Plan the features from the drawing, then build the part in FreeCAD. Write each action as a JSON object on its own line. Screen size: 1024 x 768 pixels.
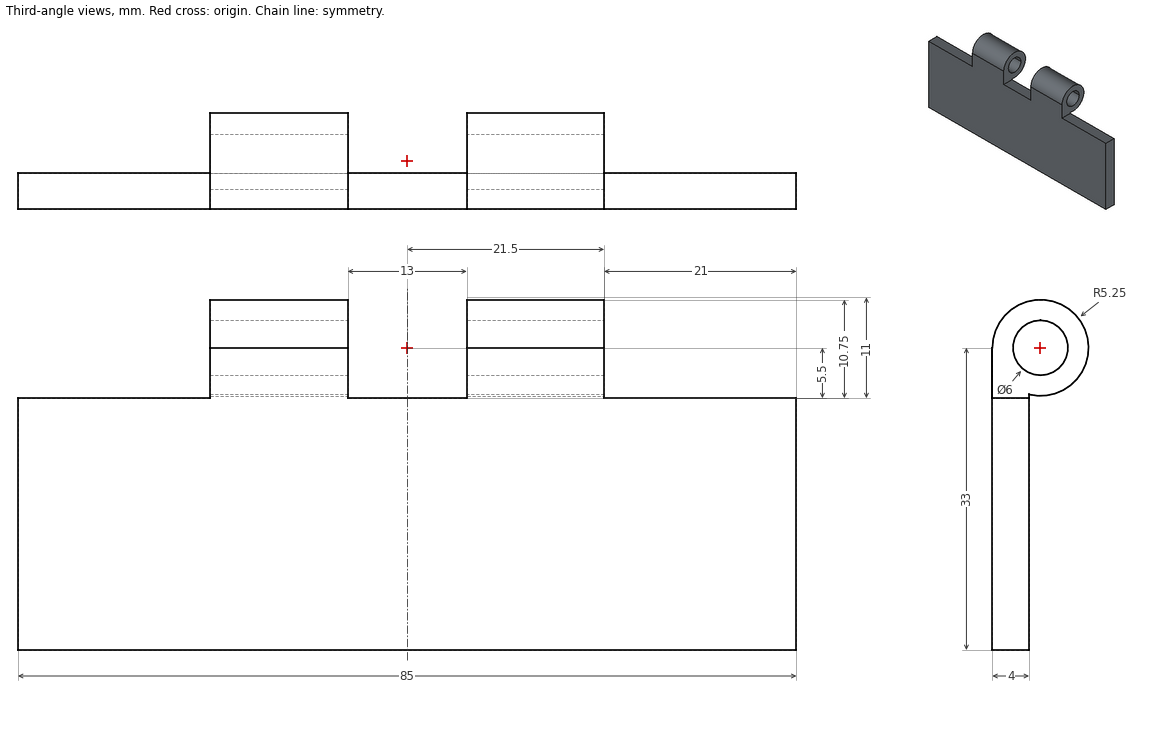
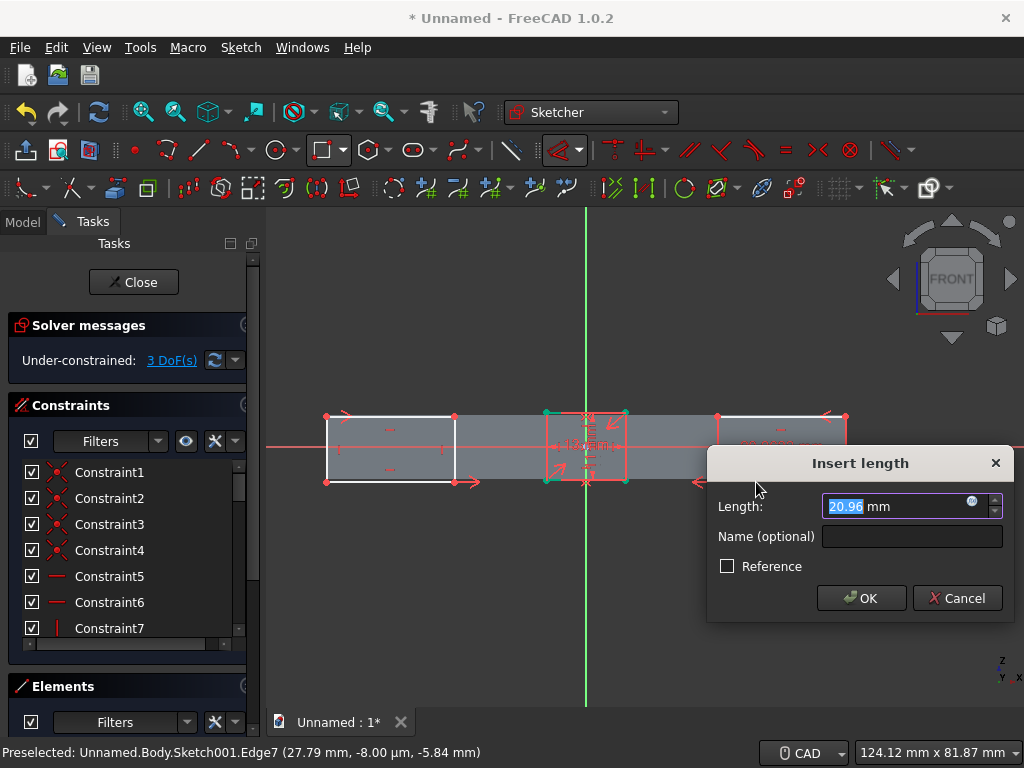
{"action": "type", "text": "21"}
{"action": "key", "text": "Return"}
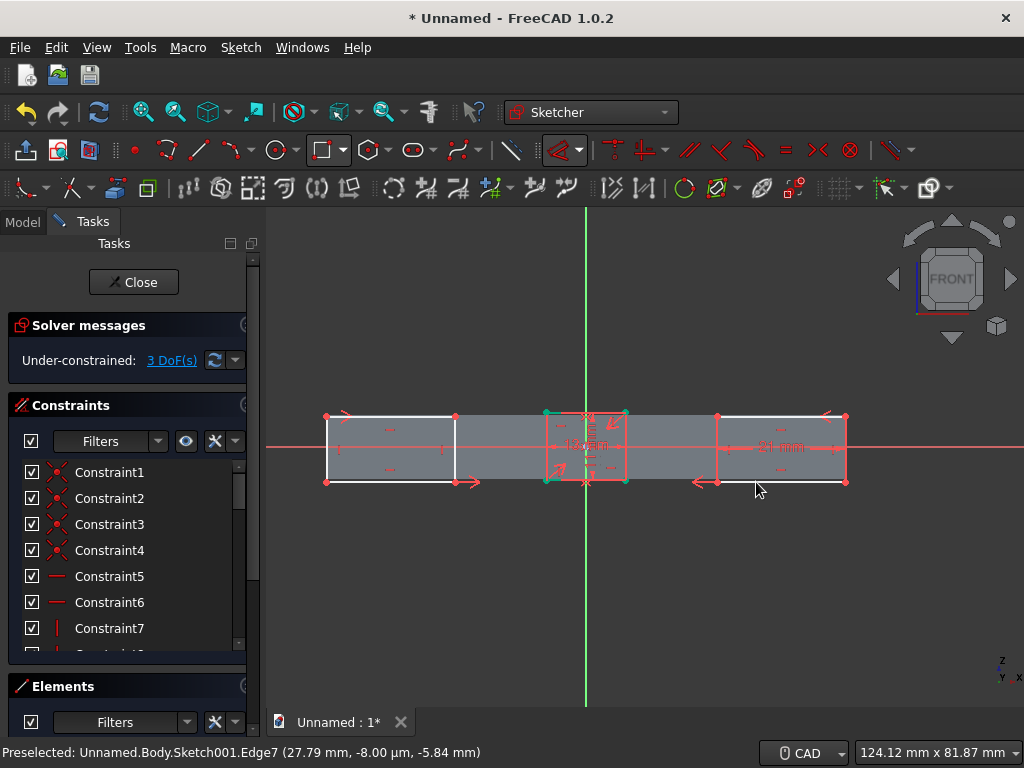
{"action": "left_click", "coordinate": [717, 482]}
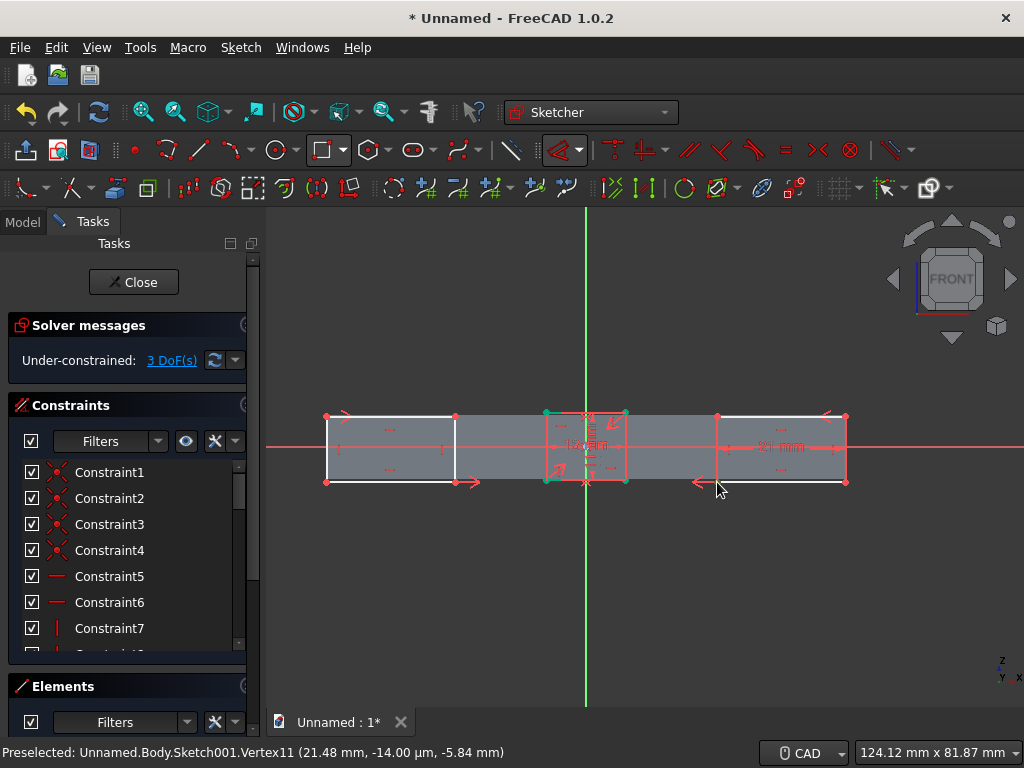
{"action": "key", "text": "i"}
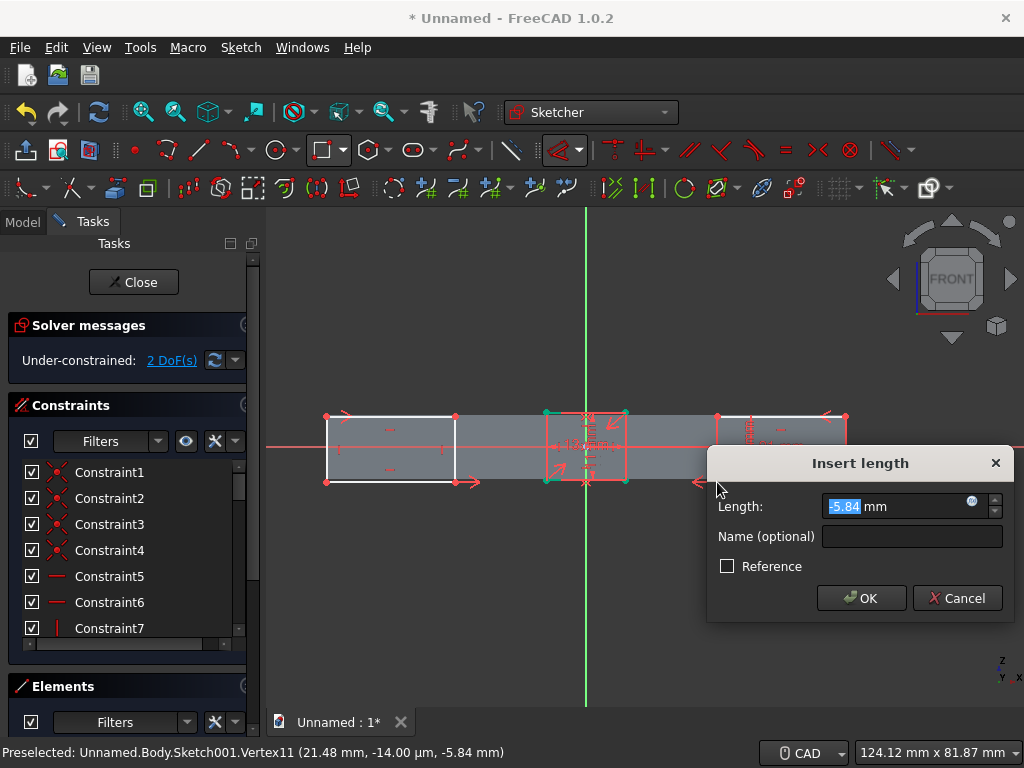
{"action": "type", "text": "-5.5"}
{"action": "key", "text": "Return"}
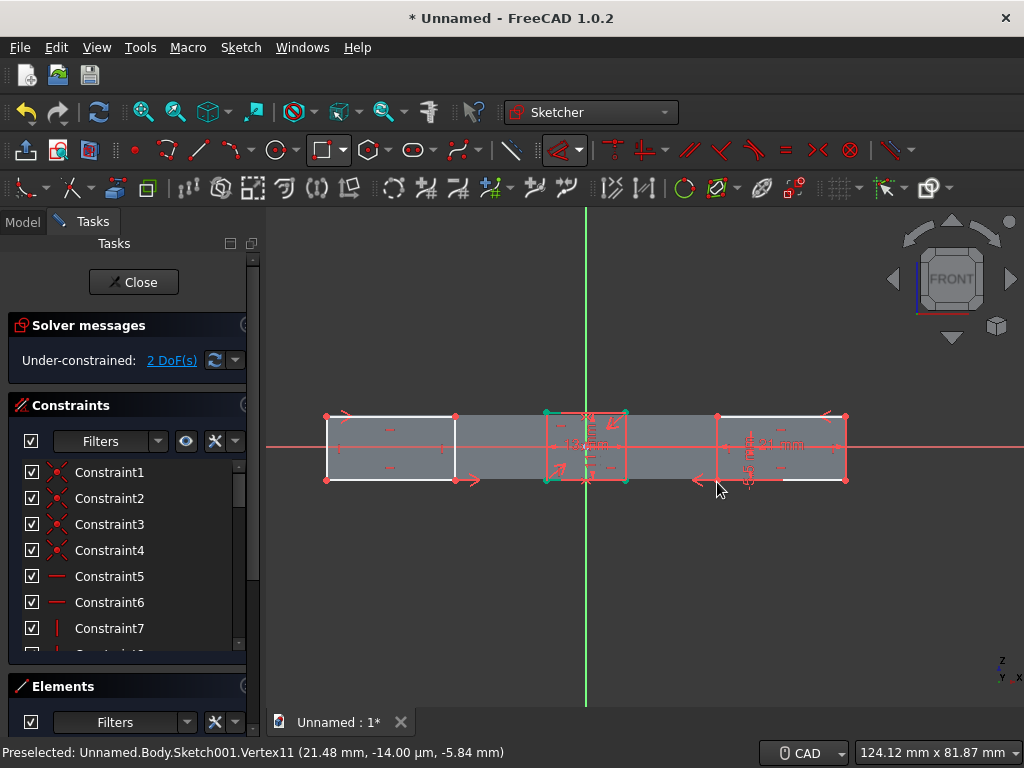
{"action": "scroll", "coordinate": [717, 436], "scroll_direction": "up", "scroll_amount": 2}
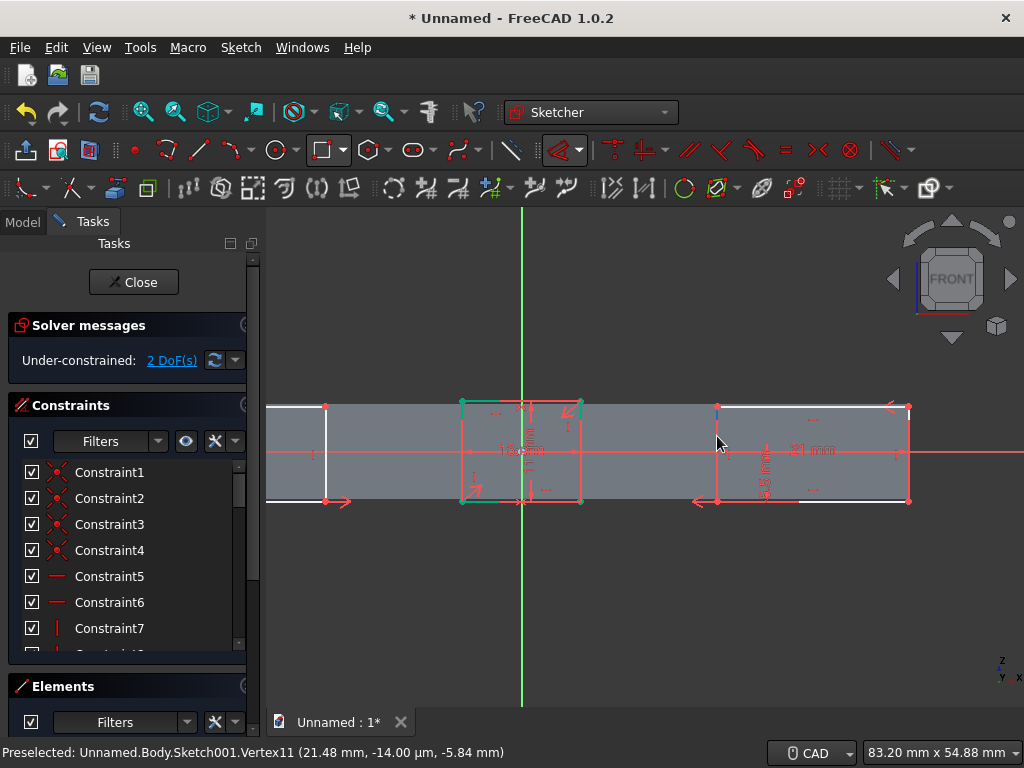
{"action": "left_click", "coordinate": [717, 435]}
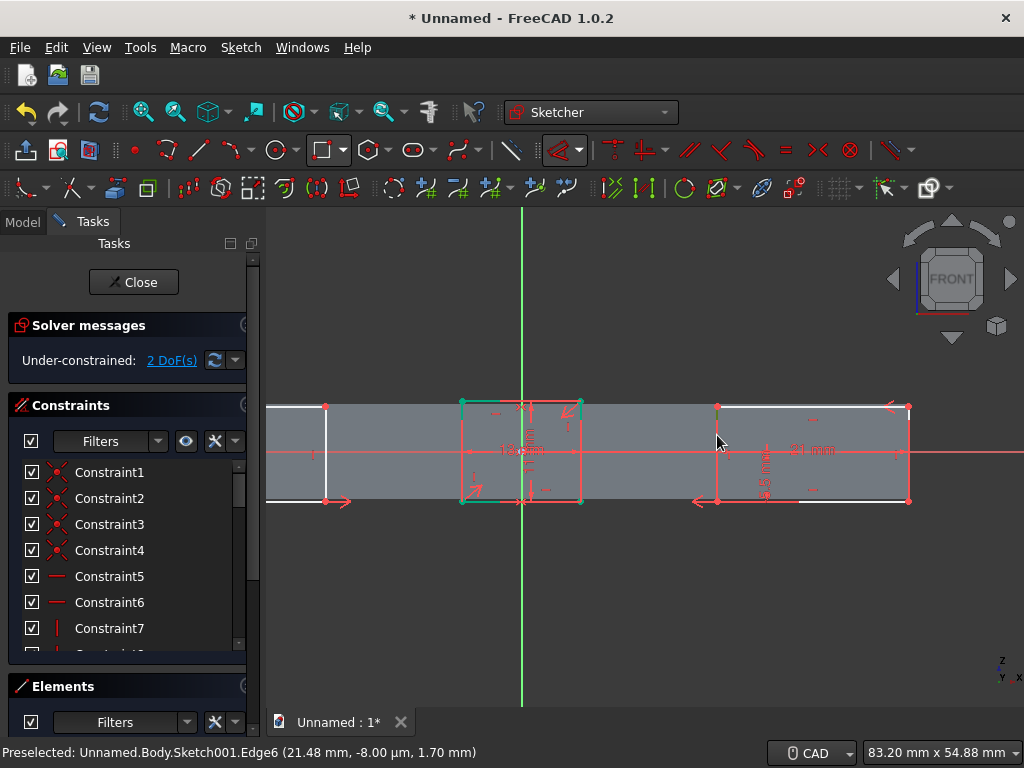
{"action": "left_click", "coordinate": [582, 150]}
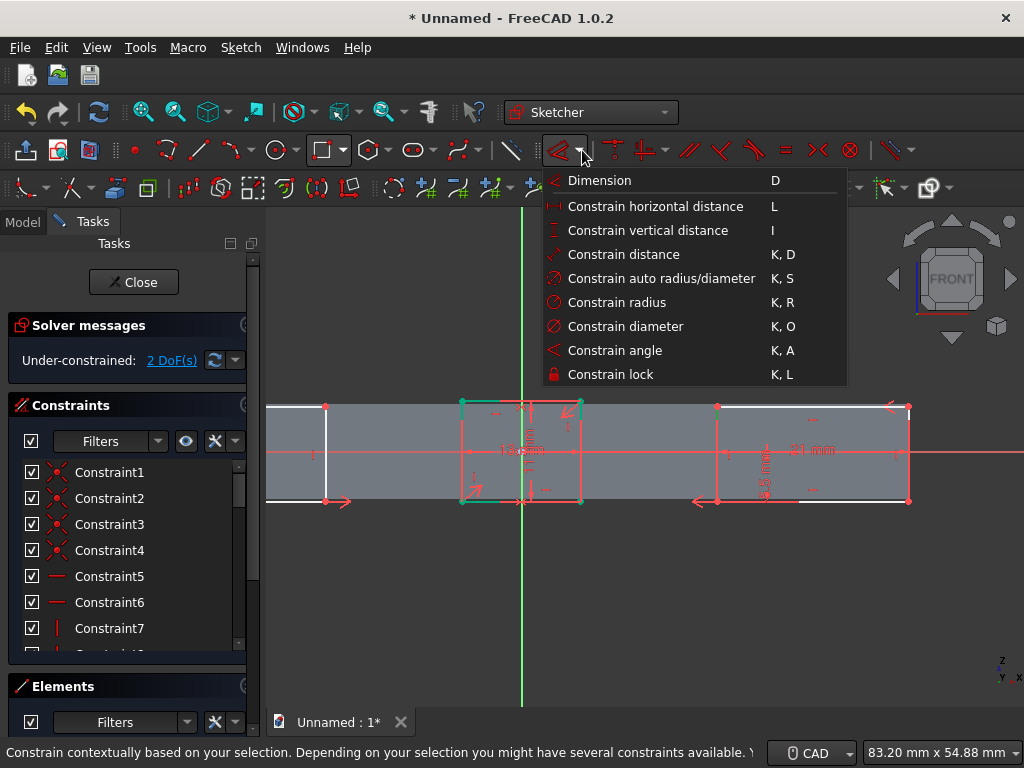
{"action": "left_click", "coordinate": [695, 230]}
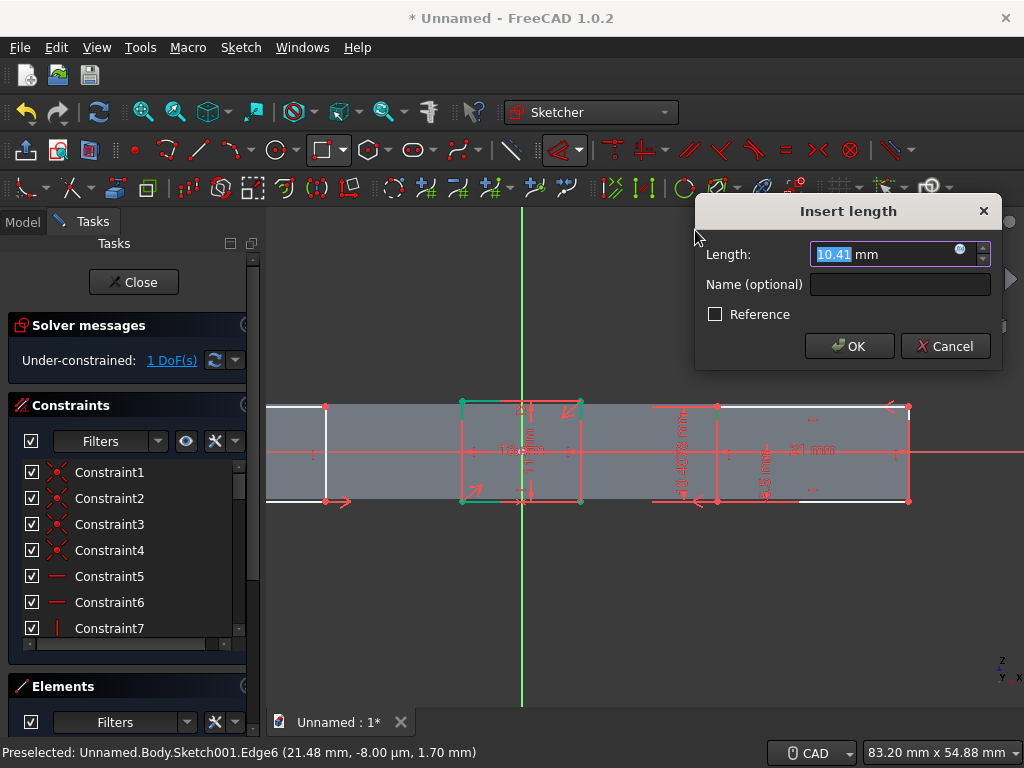
{"action": "type", "text": "10.75"}
{"action": "key", "text": "Return"}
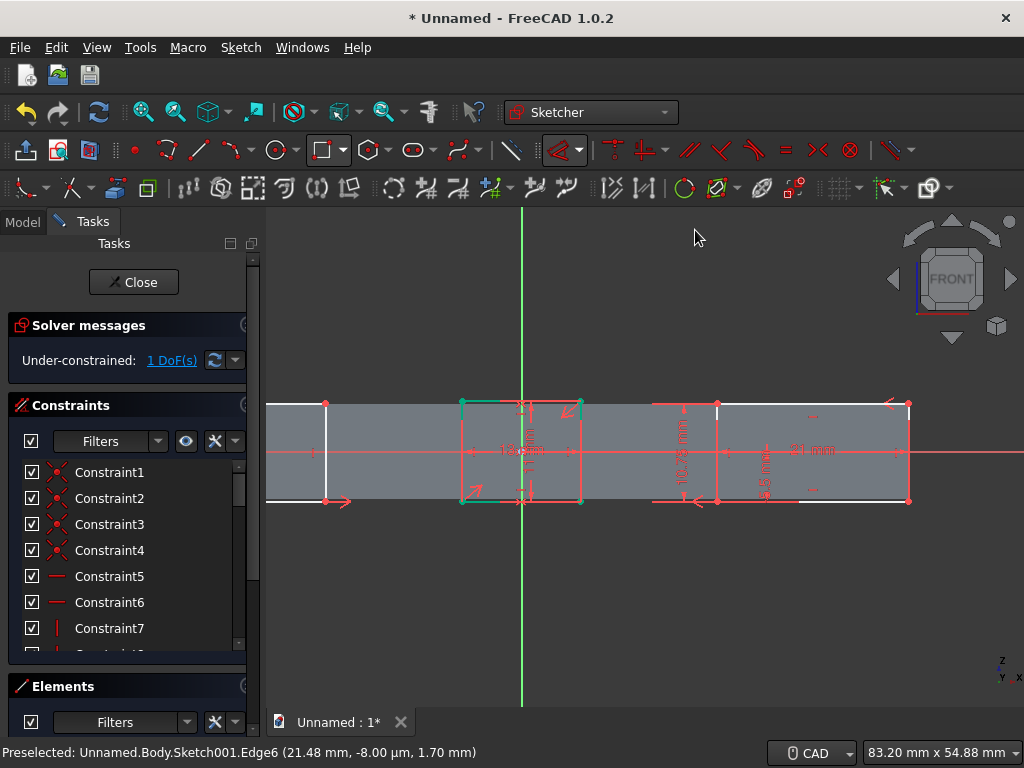
{"action": "left_click", "coordinate": [717, 404]}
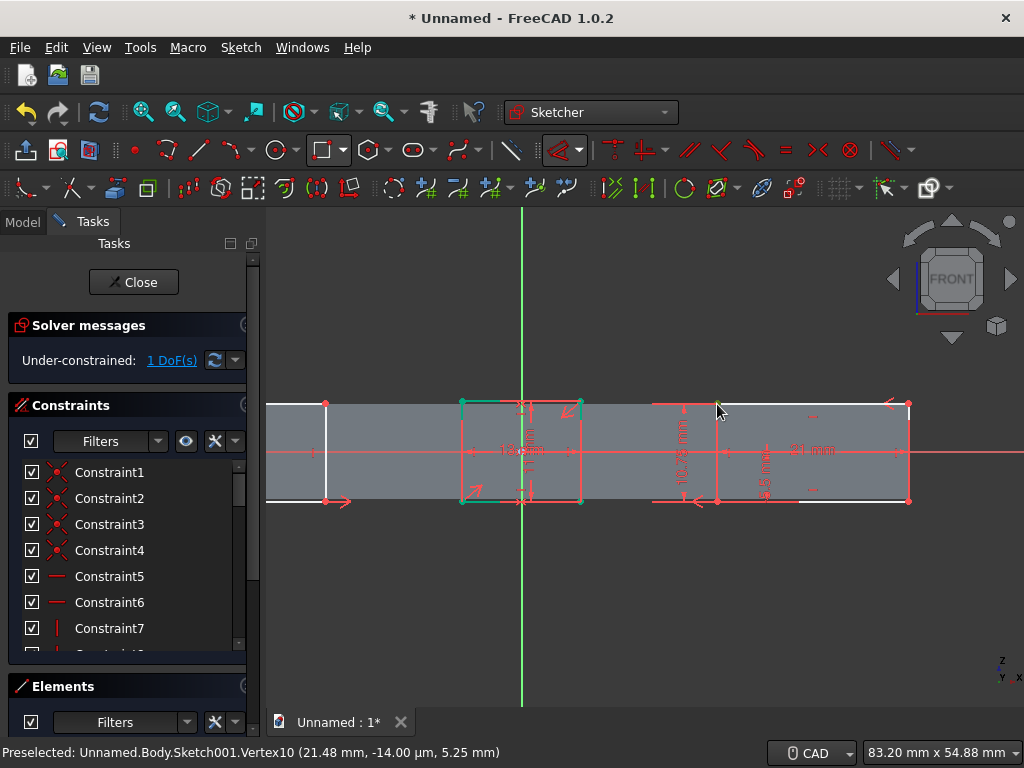
{"action": "key", "text": "l"}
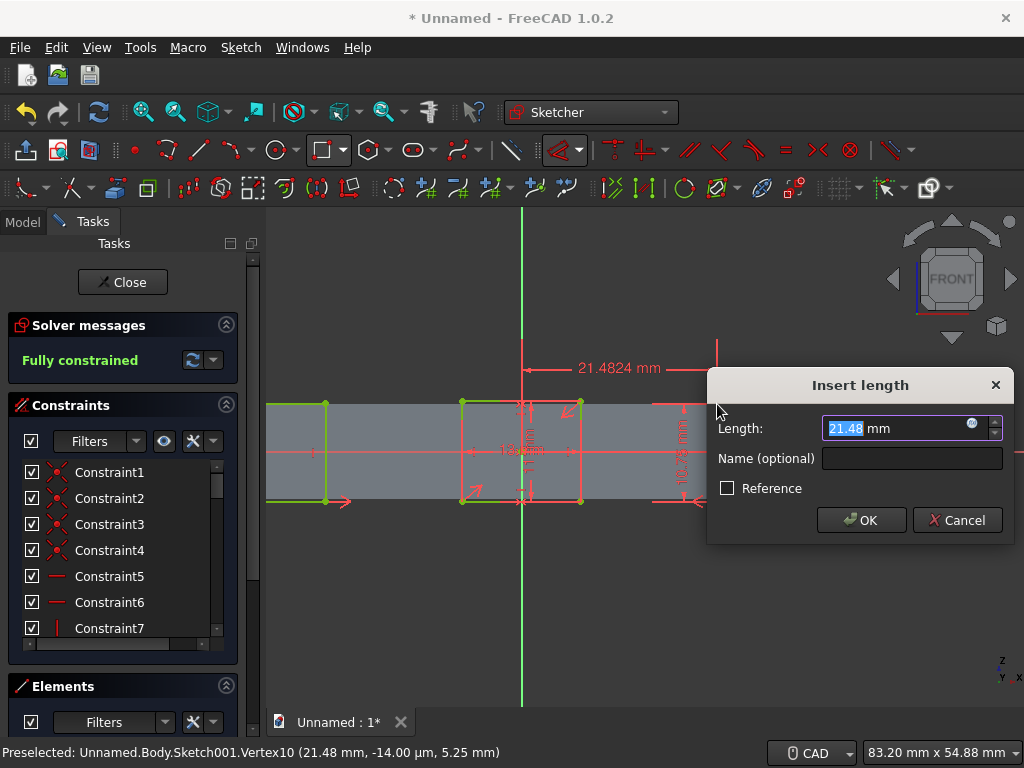
{"action": "type", "text": "21.5"}
{"action": "key", "text": "Return"}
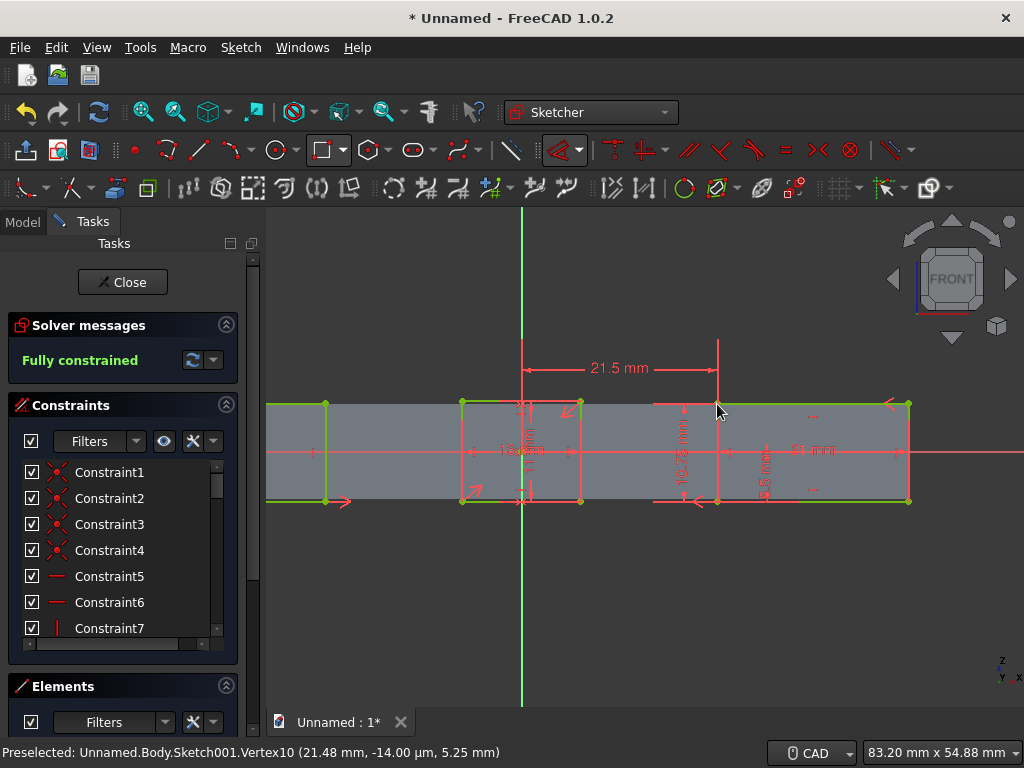
{"action": "left_click", "coordinate": [123, 282]}